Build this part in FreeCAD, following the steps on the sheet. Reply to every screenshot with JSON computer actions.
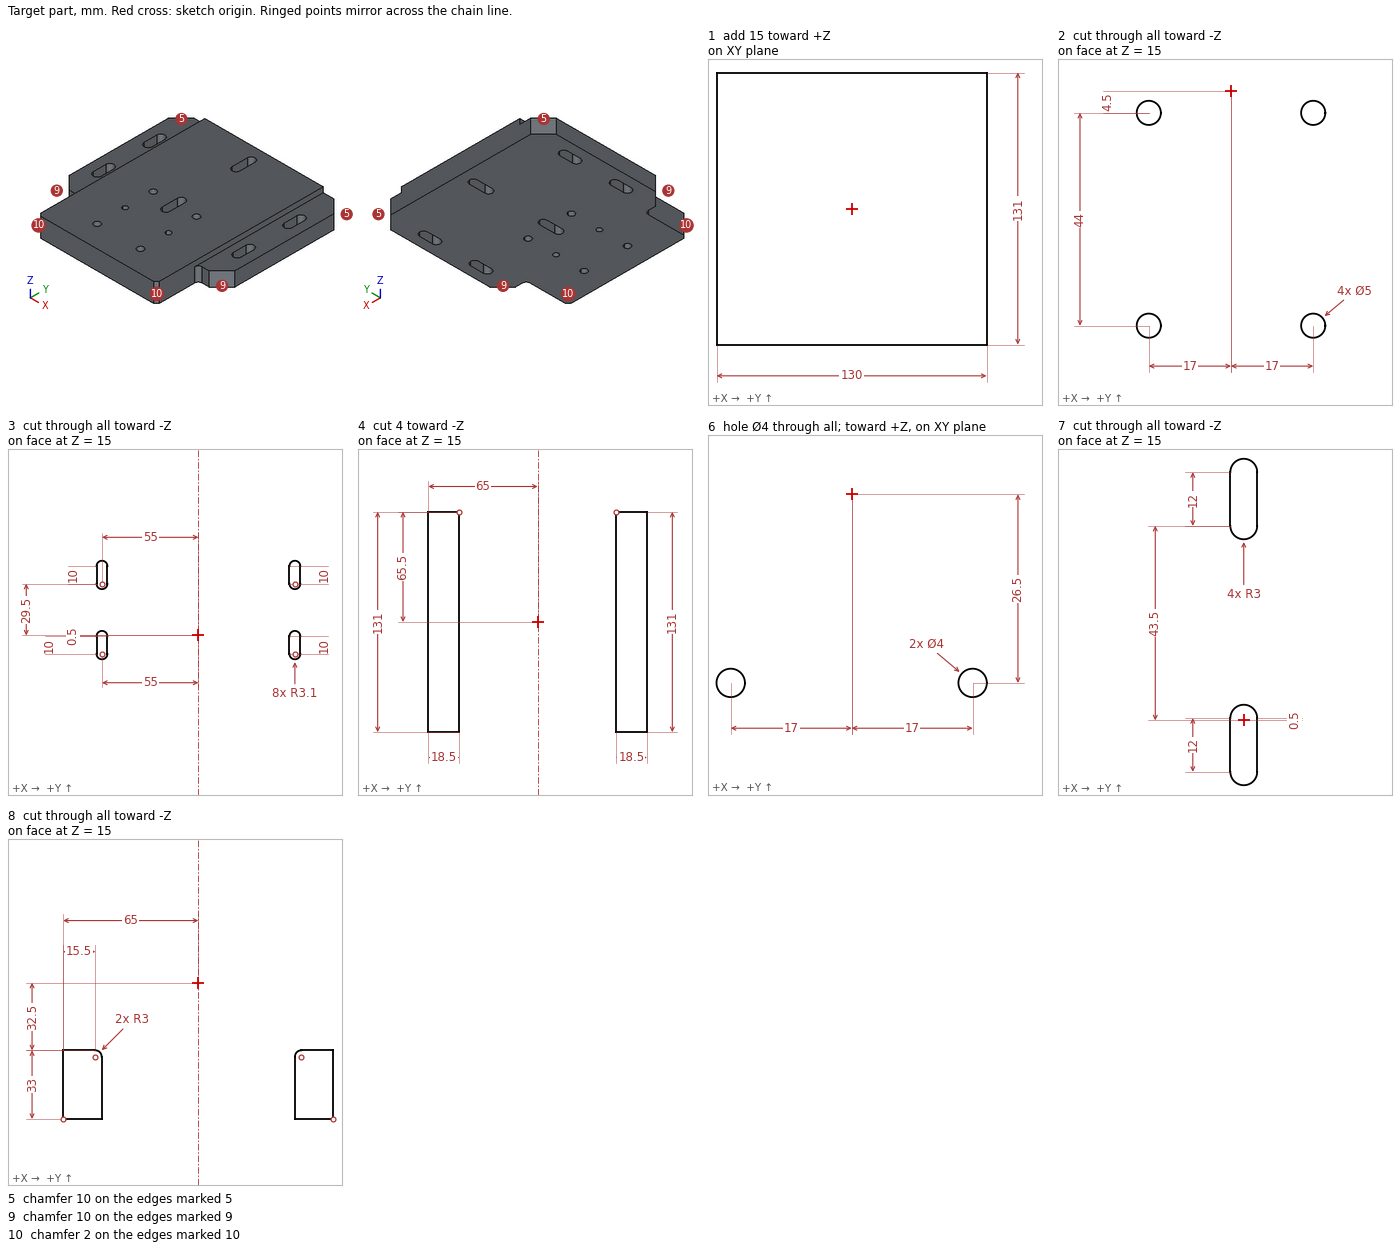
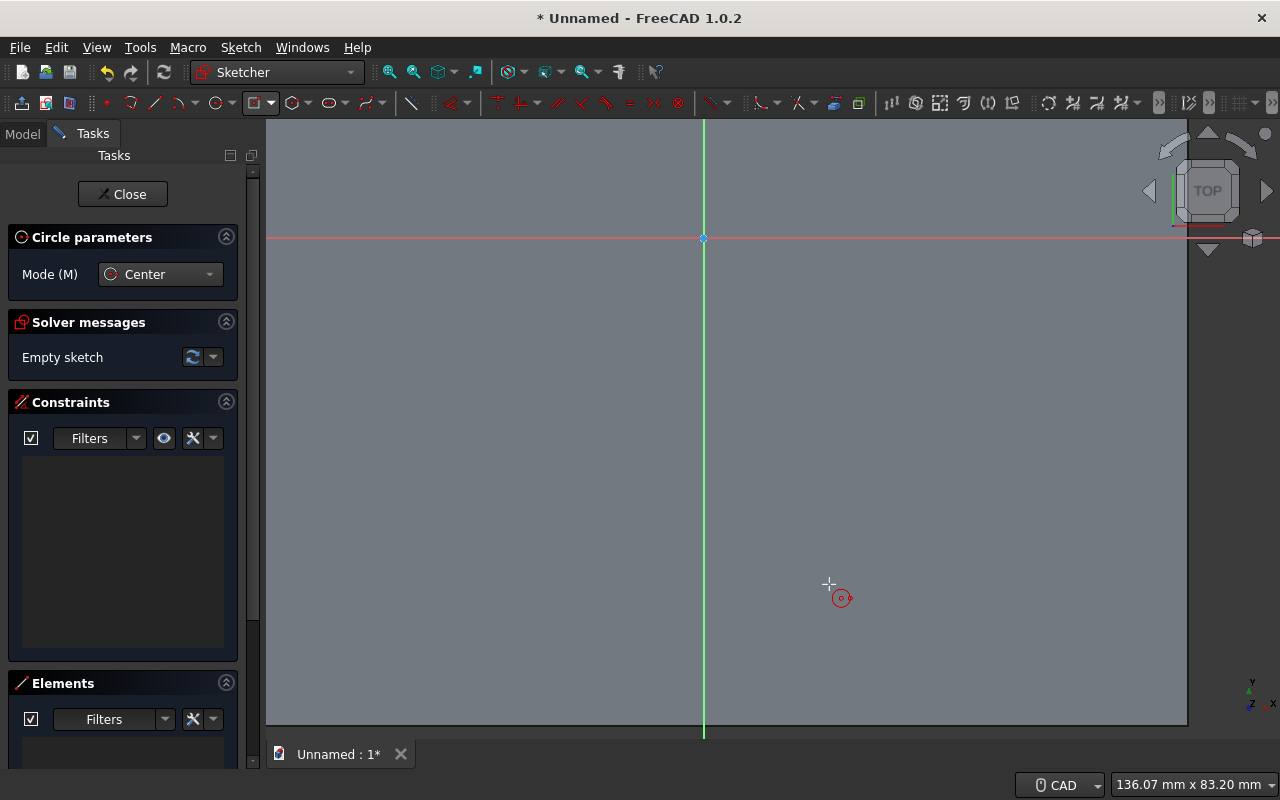
{"action": "left_click", "coordinate": [830, 600]}
{"action": "mouse_move", "coordinate": [844, 586]}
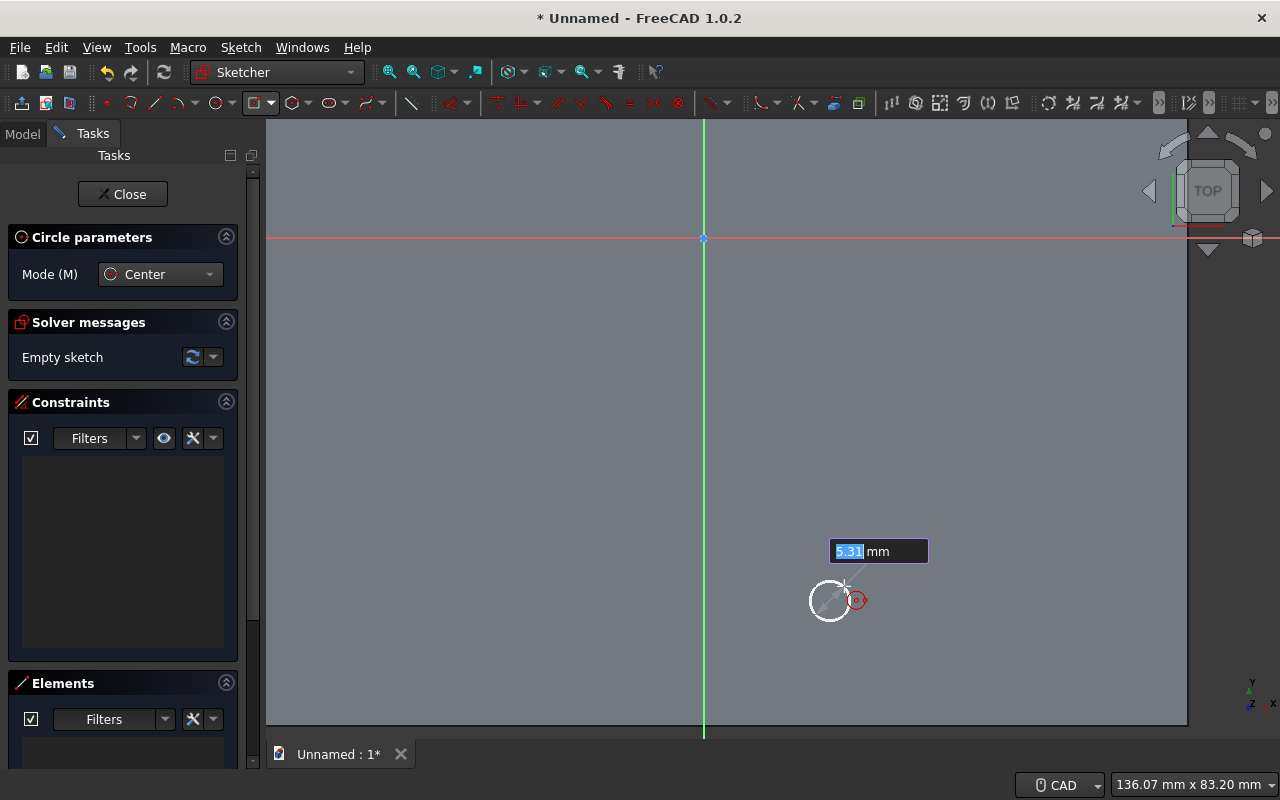
{"action": "type", "text": "5"}
{"action": "key", "text": "Return"}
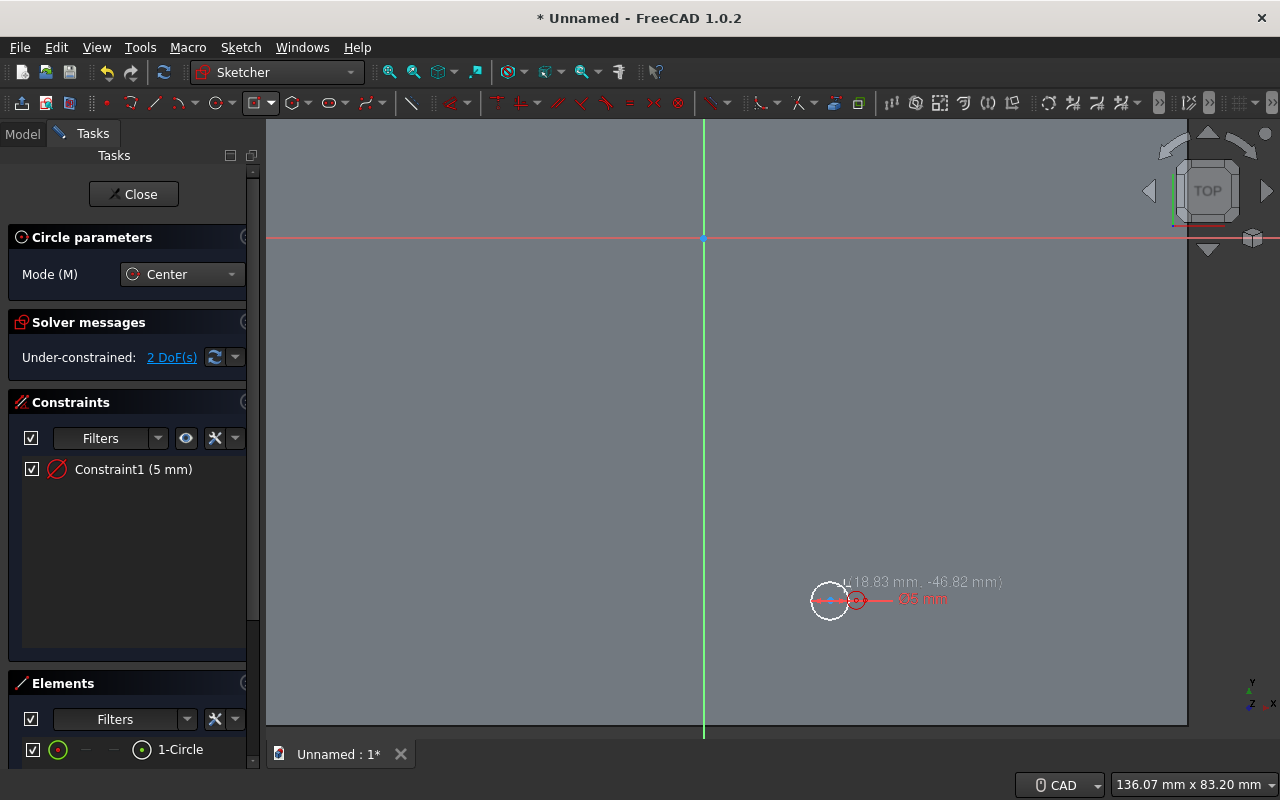
{"action": "left_click", "coordinate": [577, 600]}
{"action": "mouse_move", "coordinate": [590, 586]}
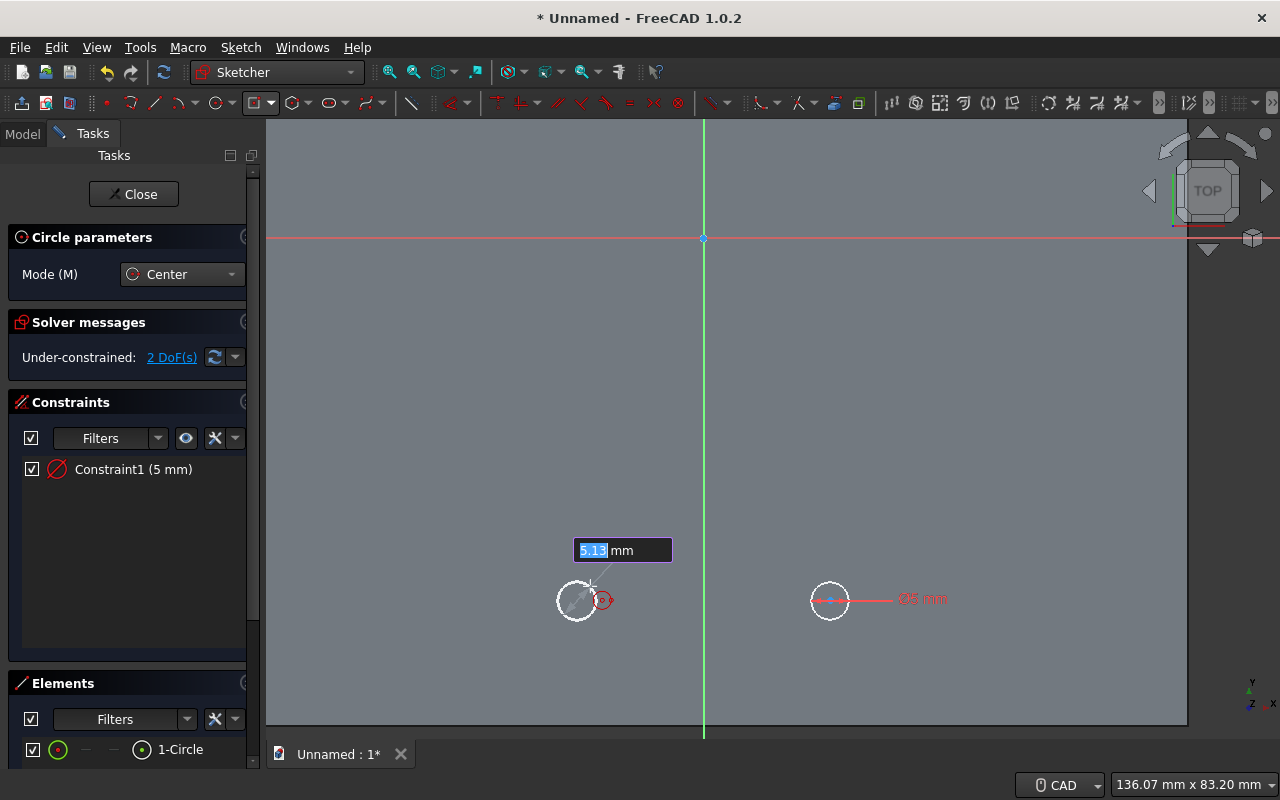
{"action": "type", "text": "5"}
{"action": "key", "text": "Return"}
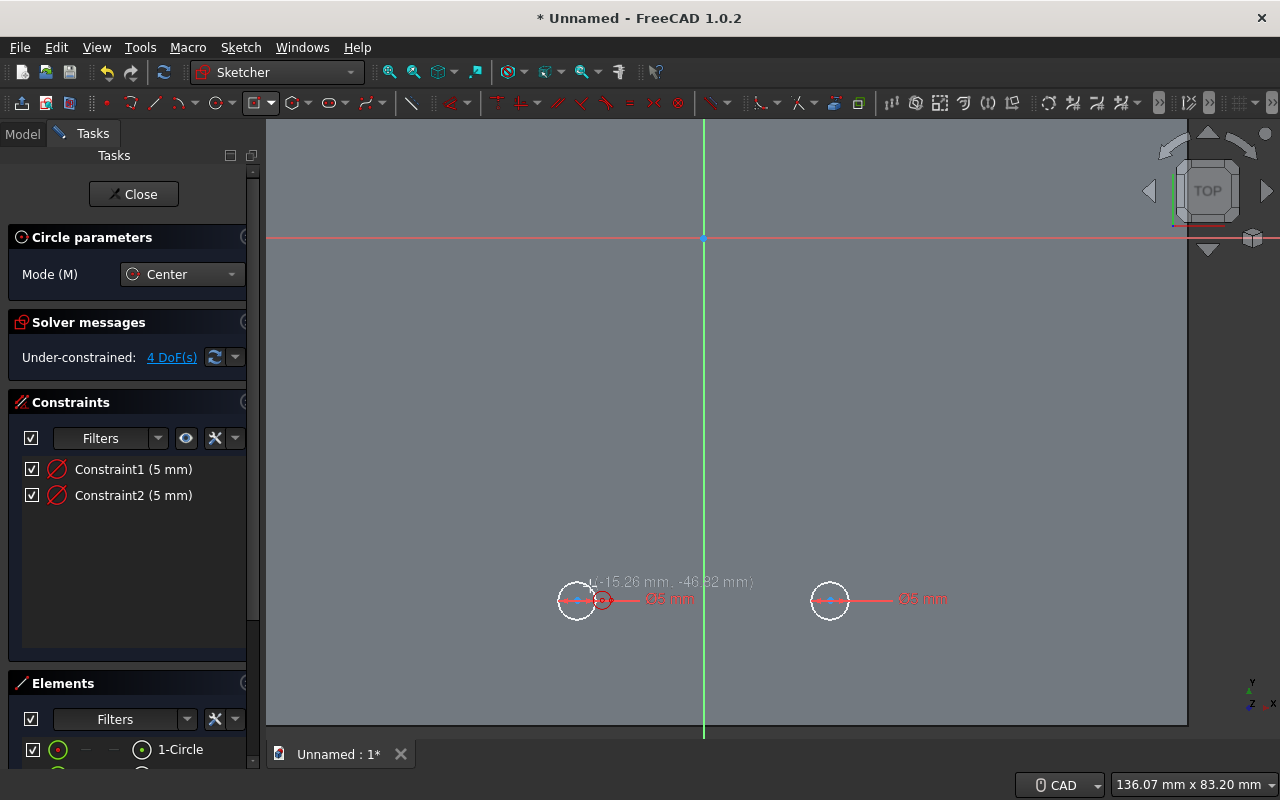
{"action": "left_click", "coordinate": [577, 272]}
{"action": "mouse_move", "coordinate": [590, 258]}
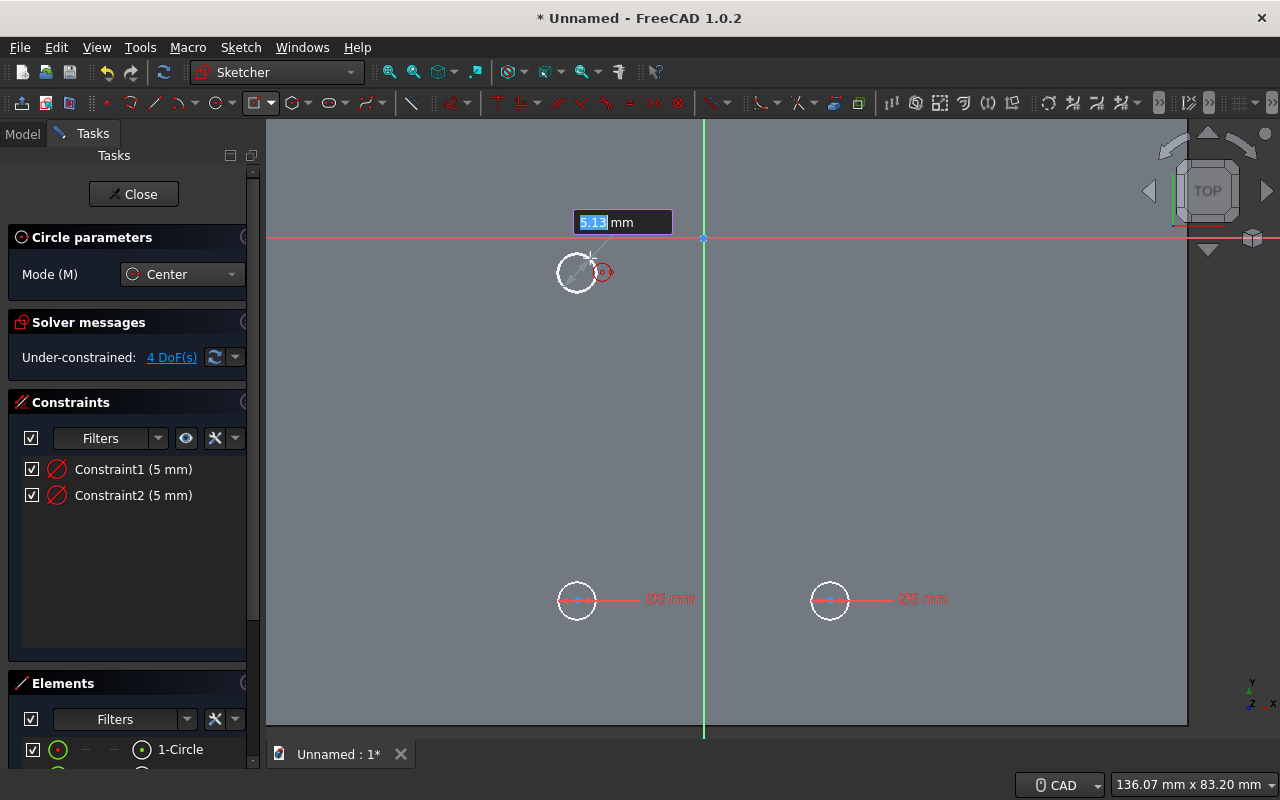
{"action": "type", "text": "5"}
{"action": "key", "text": "Return"}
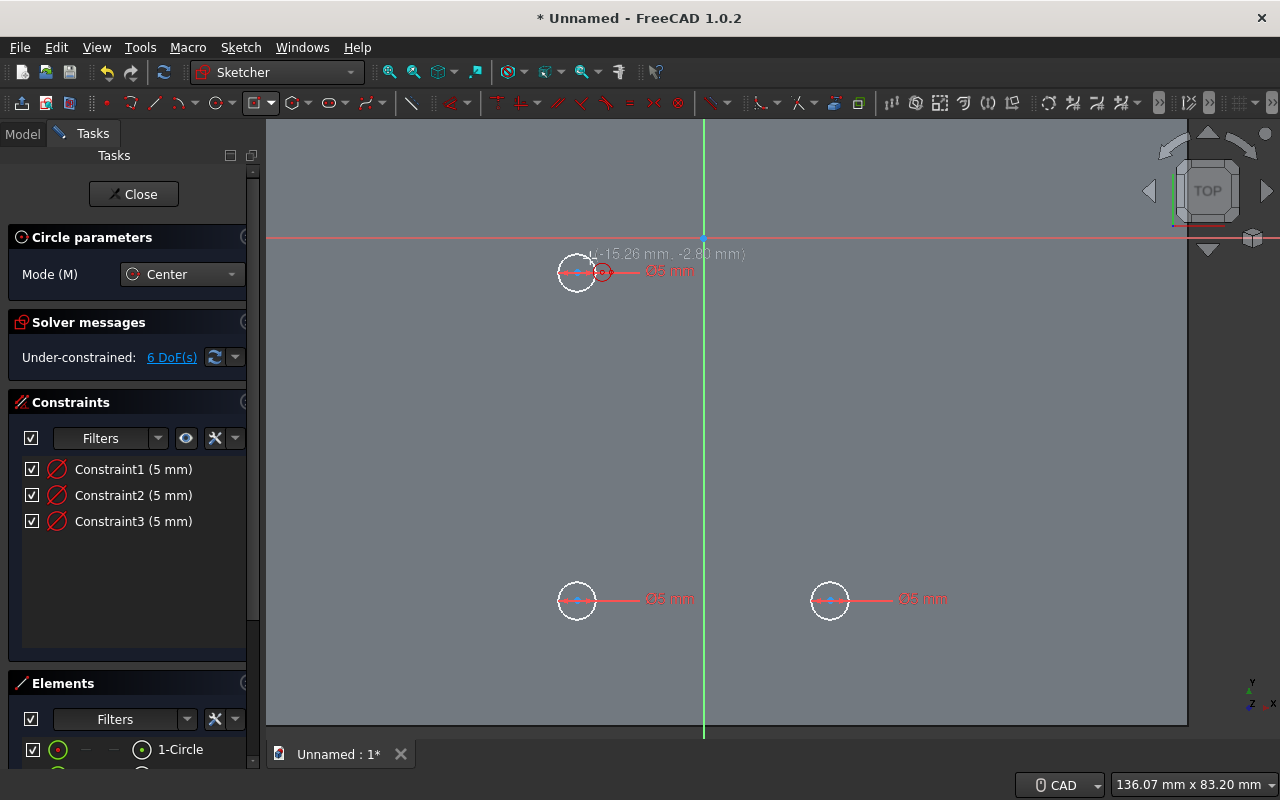
{"action": "left_click", "coordinate": [830, 272]}
{"action": "mouse_move", "coordinate": [844, 258]}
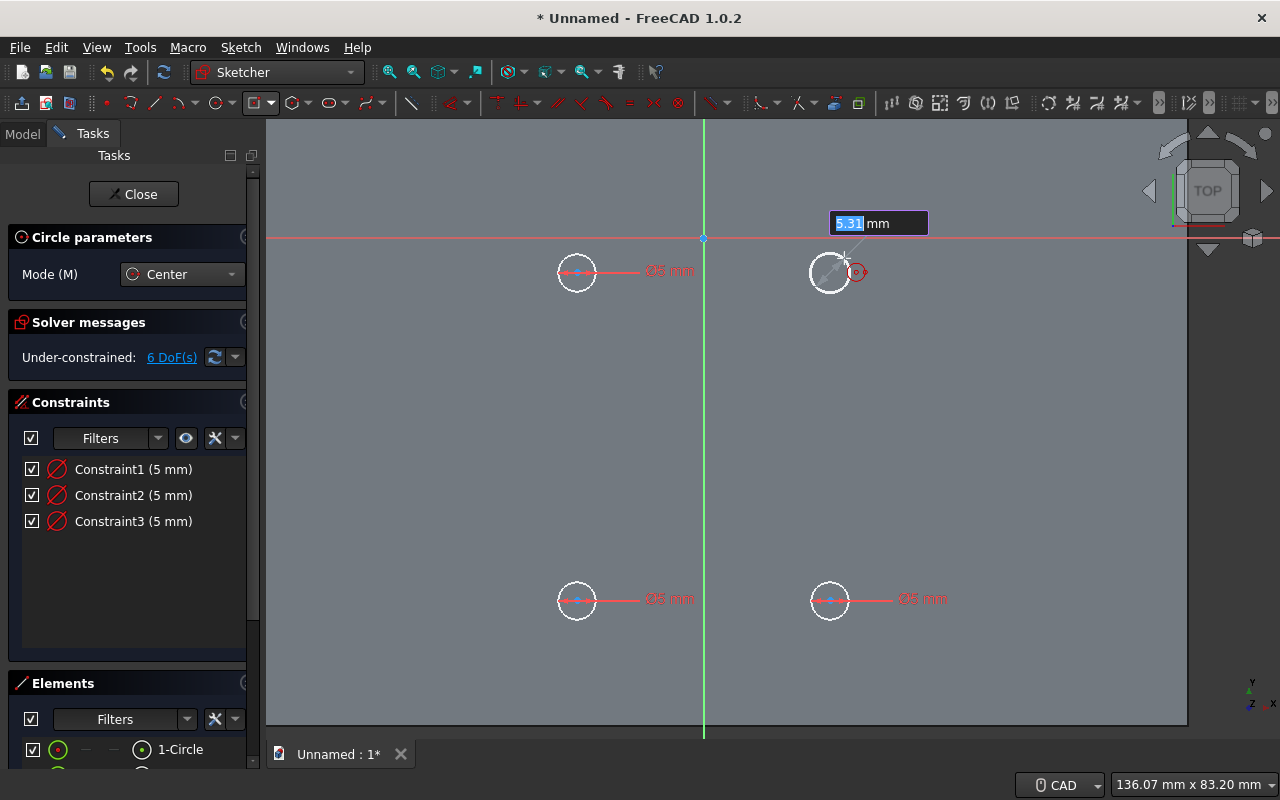
{"action": "type", "text": "5"}
{"action": "key", "text": "Return"}
{"action": "key", "text": "Escape"}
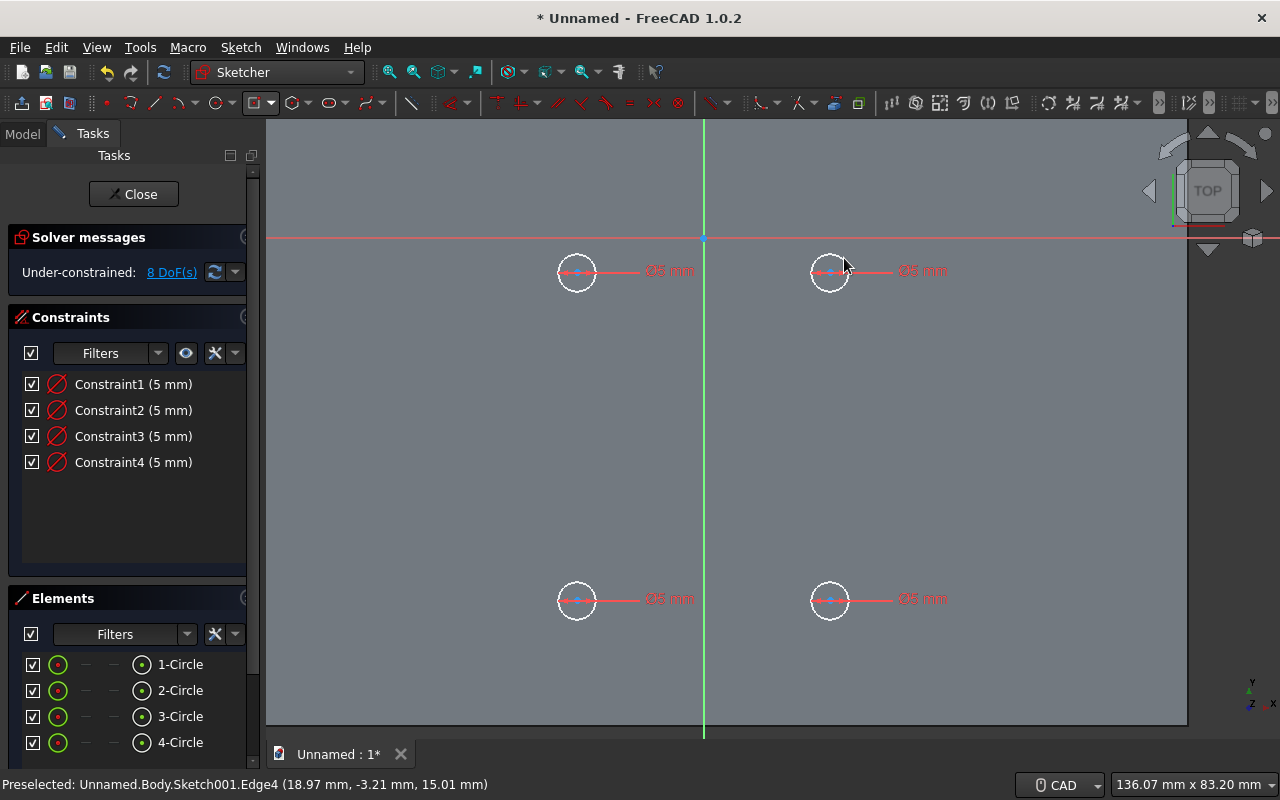
{"action": "left_click", "coordinate": [830, 601]}